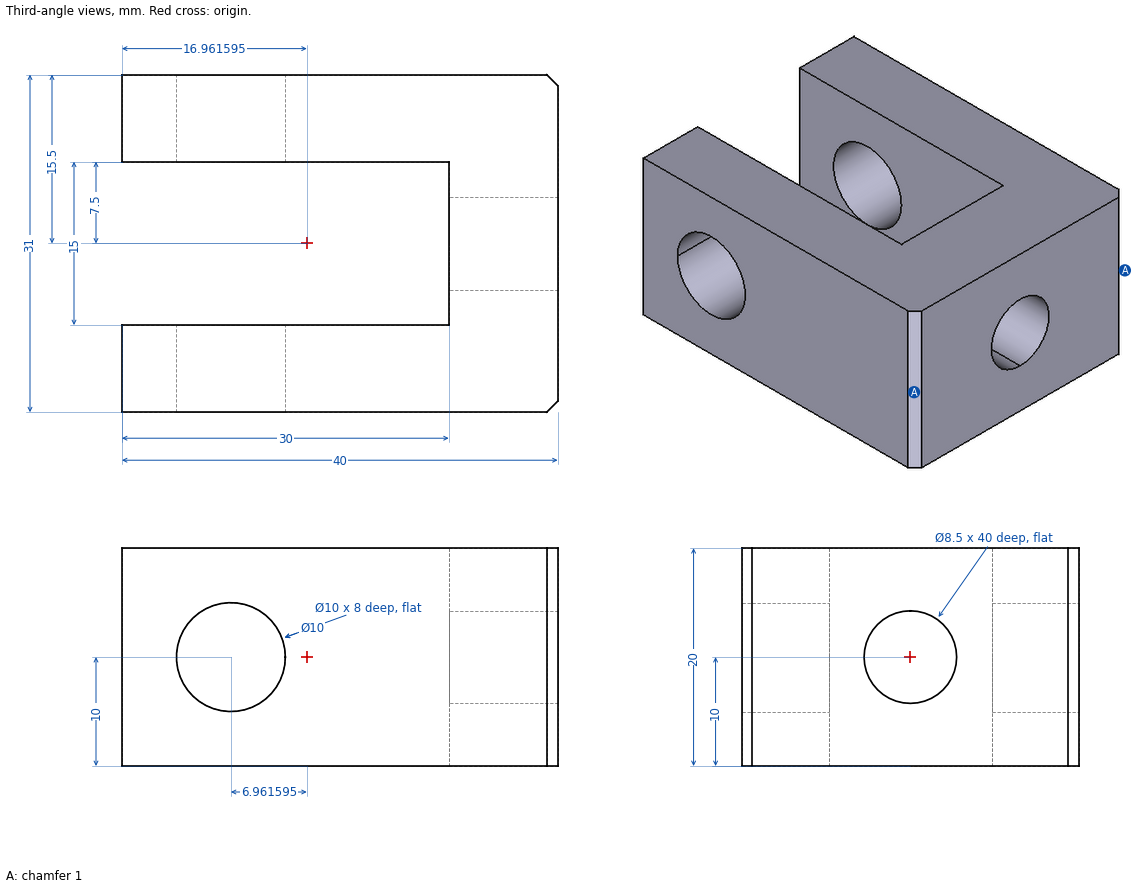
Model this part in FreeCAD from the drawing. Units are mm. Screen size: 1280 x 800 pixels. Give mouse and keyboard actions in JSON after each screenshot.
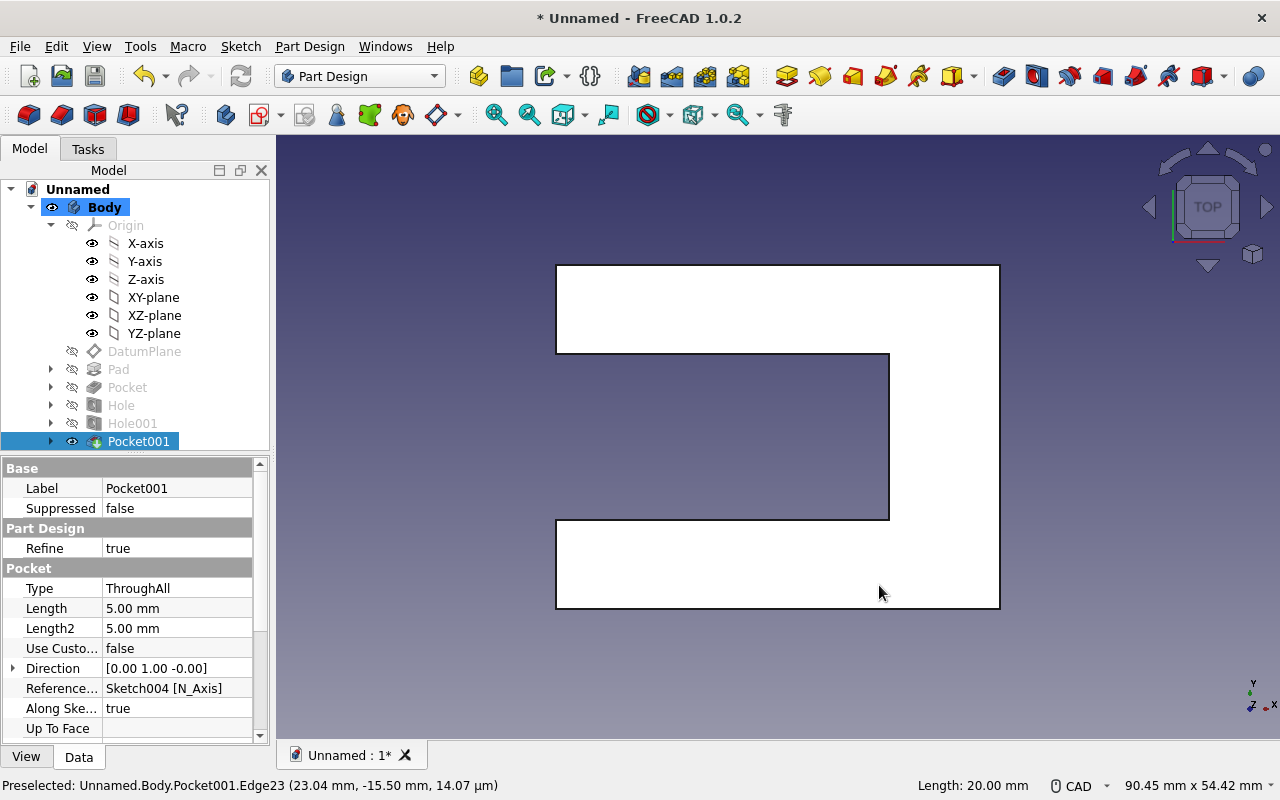
{"action": "key", "text": "1"}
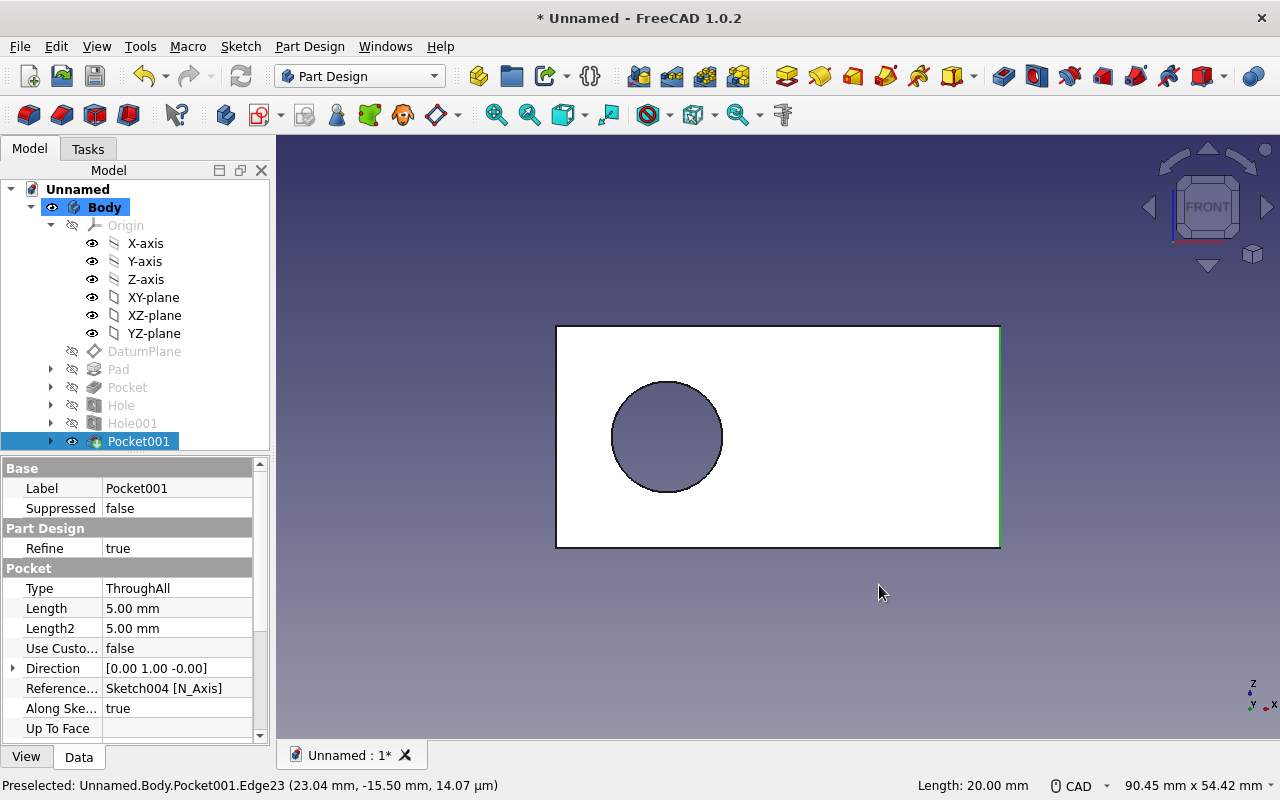
{"action": "left_click", "coordinate": [497, 116]}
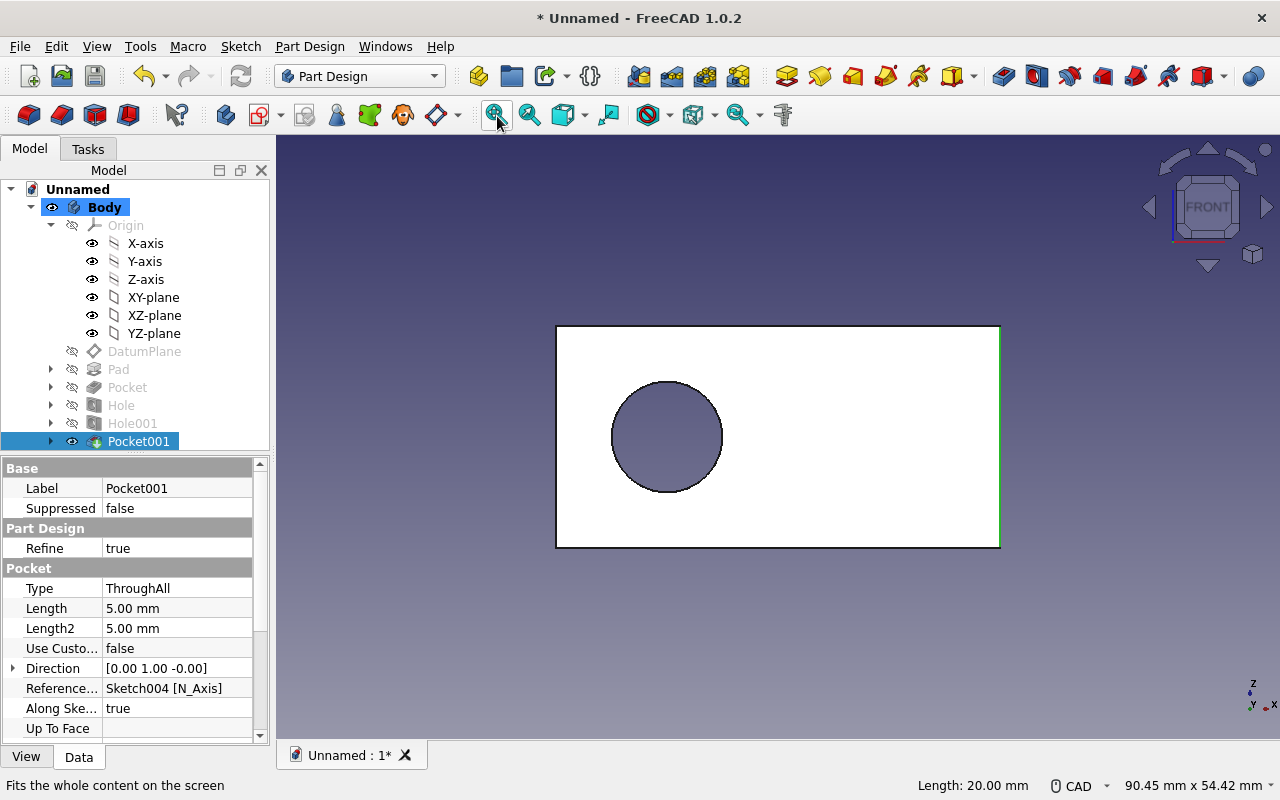
{"action": "key", "text": "3"}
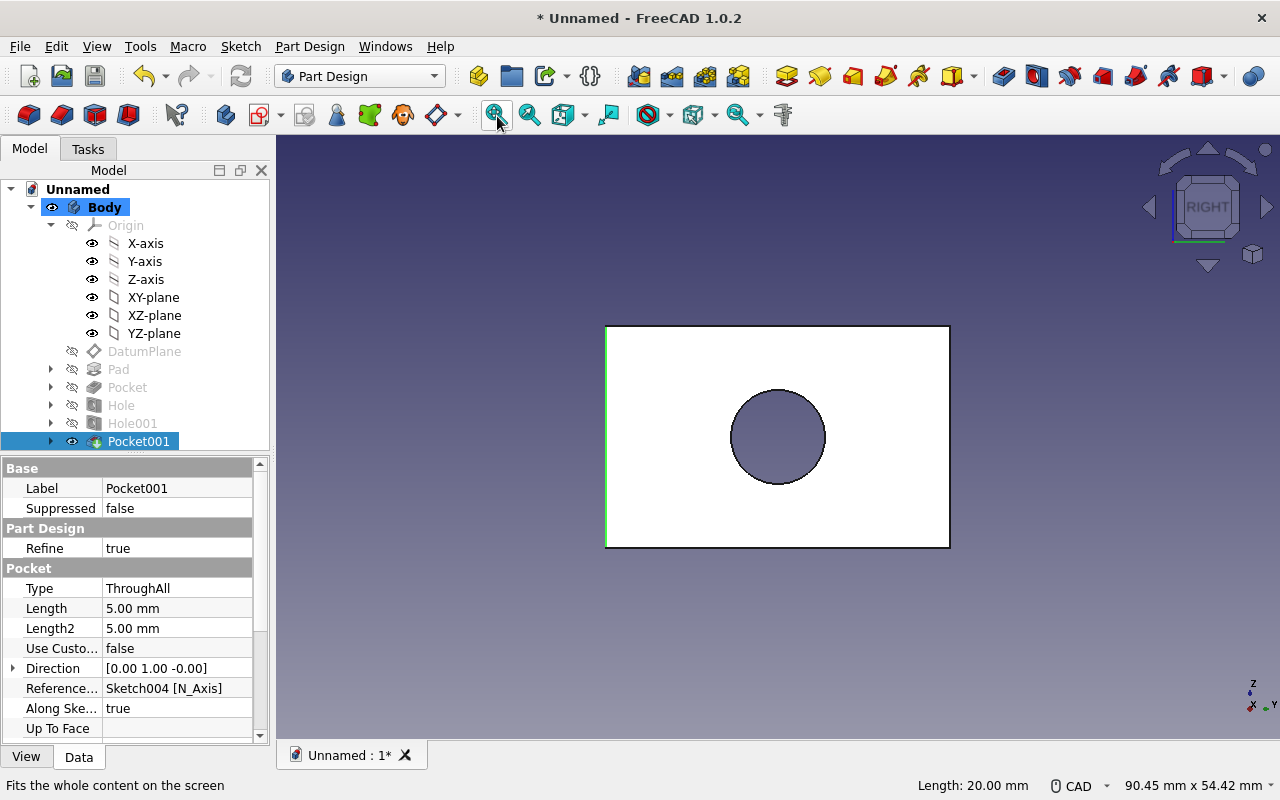
{"action": "key", "text": "v f"}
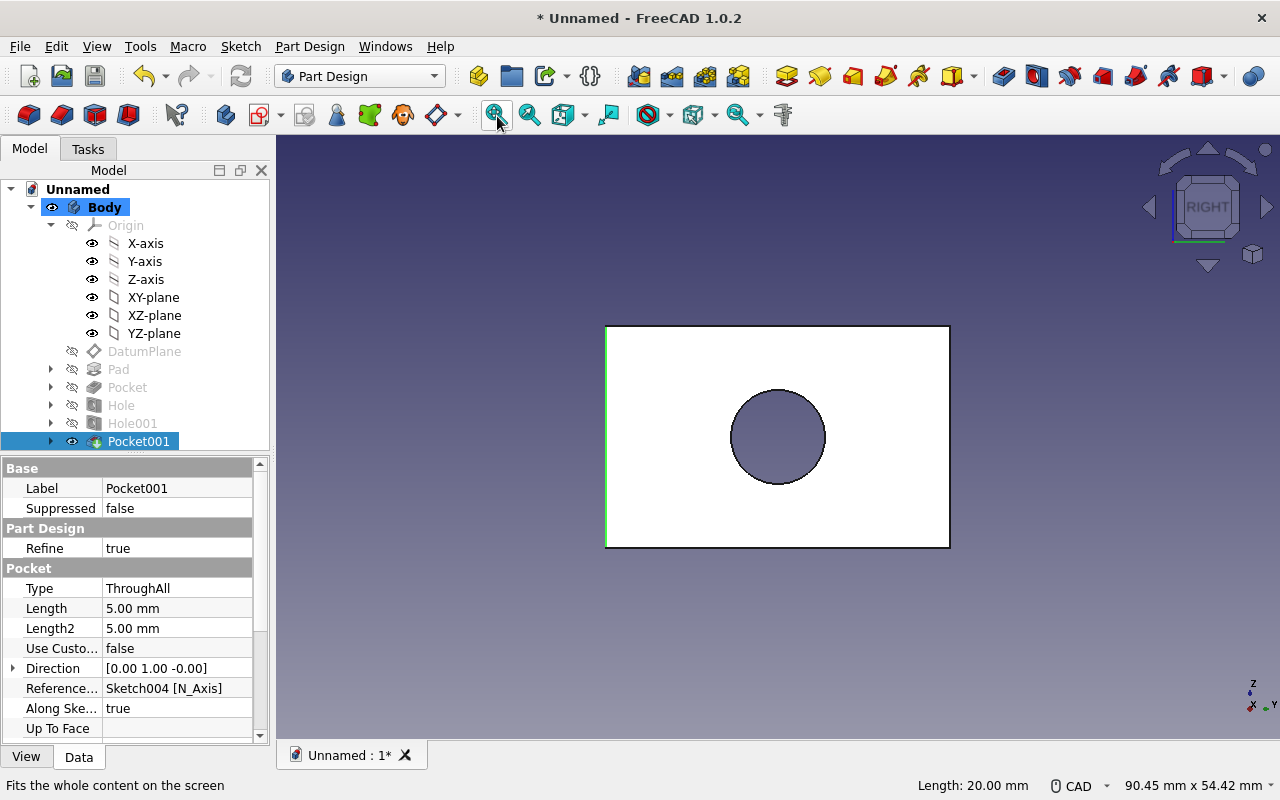
{"action": "left_click", "coordinate": [950, 436], "text": "ctrl"}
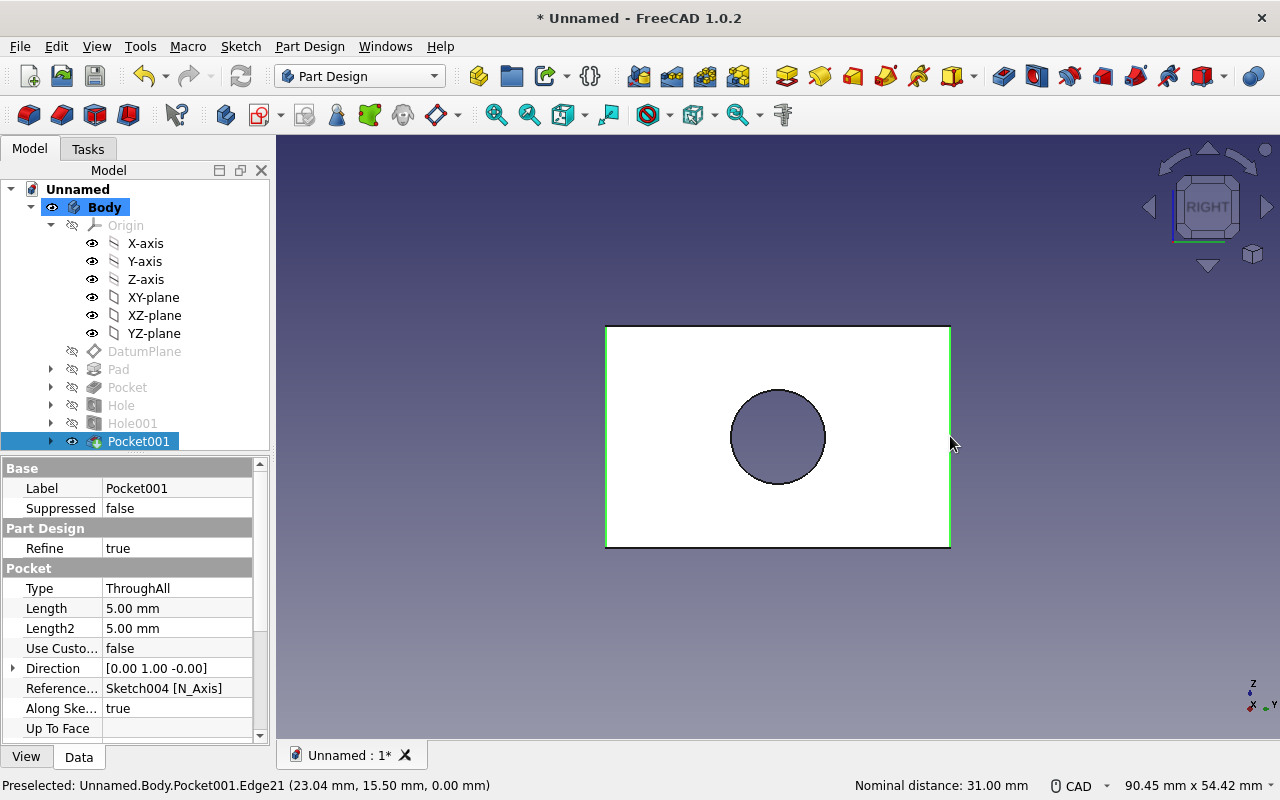
{"action": "left_click", "coordinate": [62, 116]}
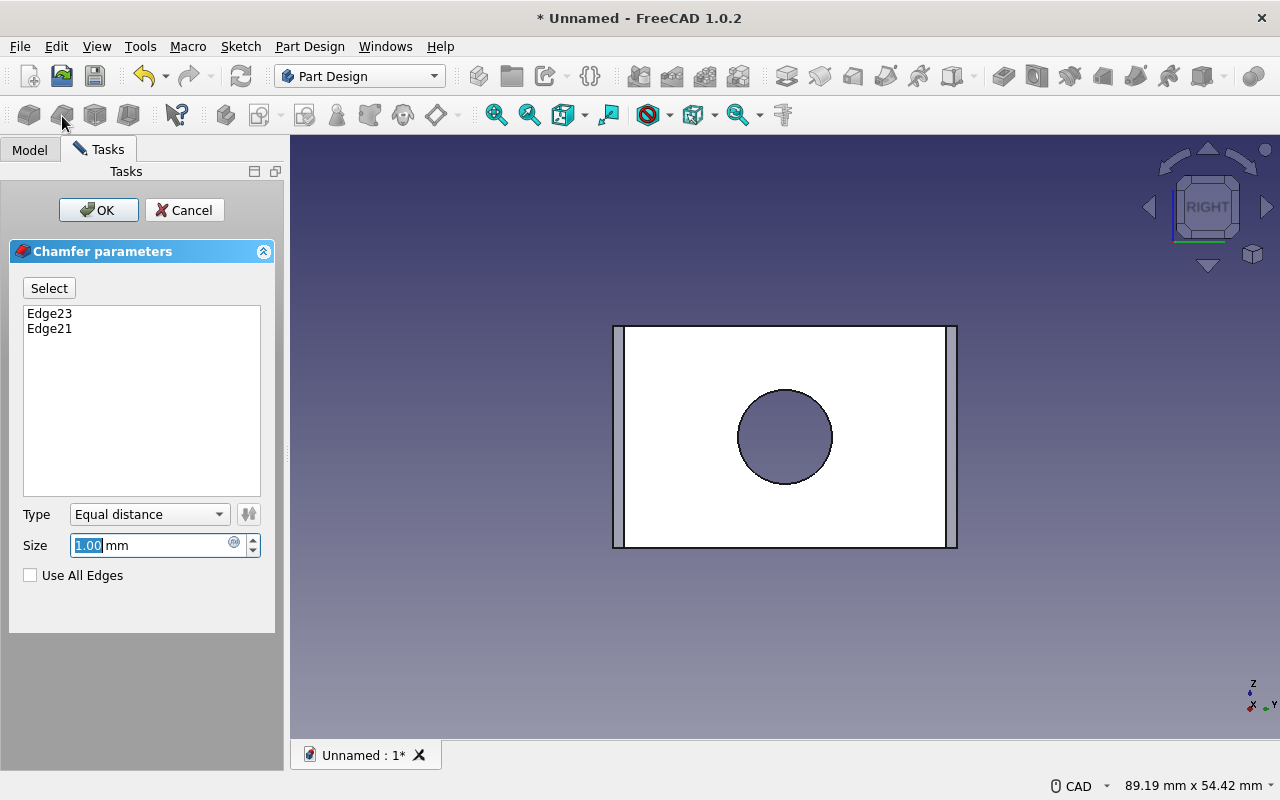
{"action": "type", "text": "1"}
{"action": "key", "text": "Tab"}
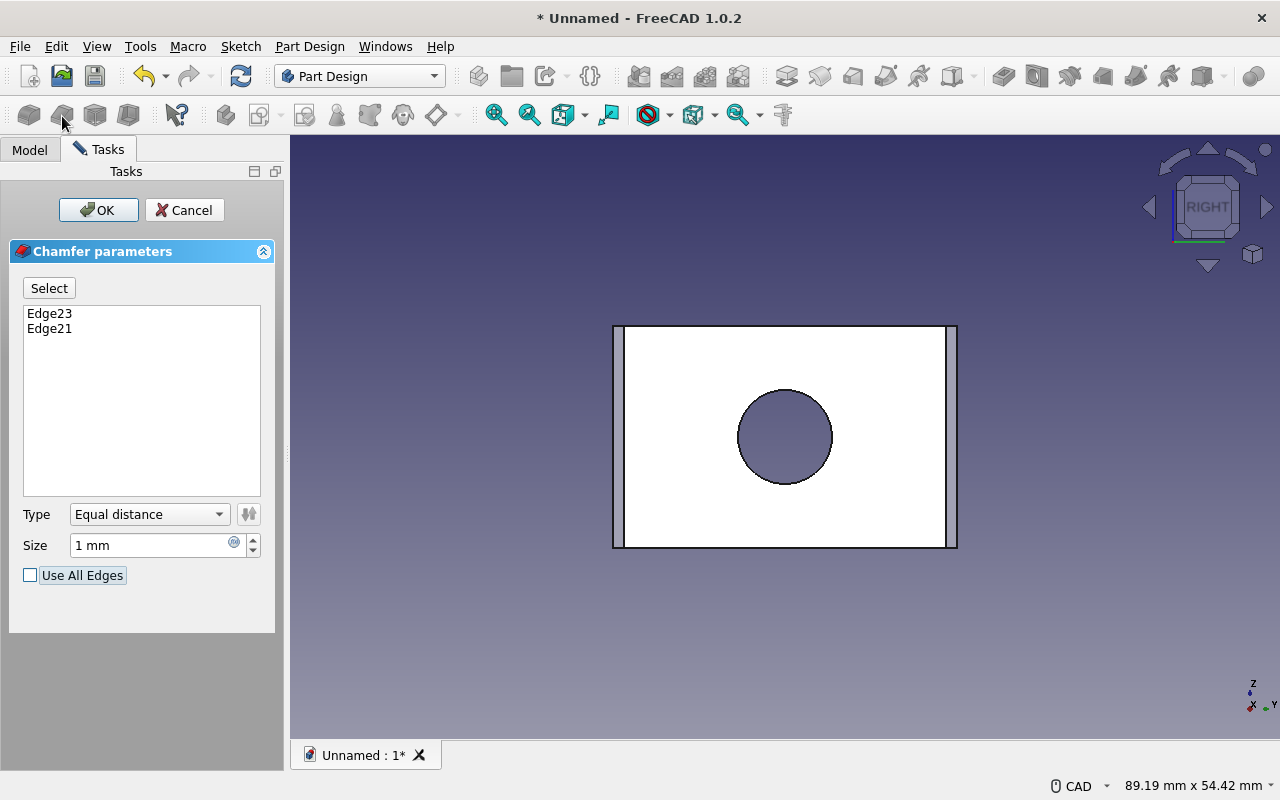
{"action": "left_click", "coordinate": [99, 210]}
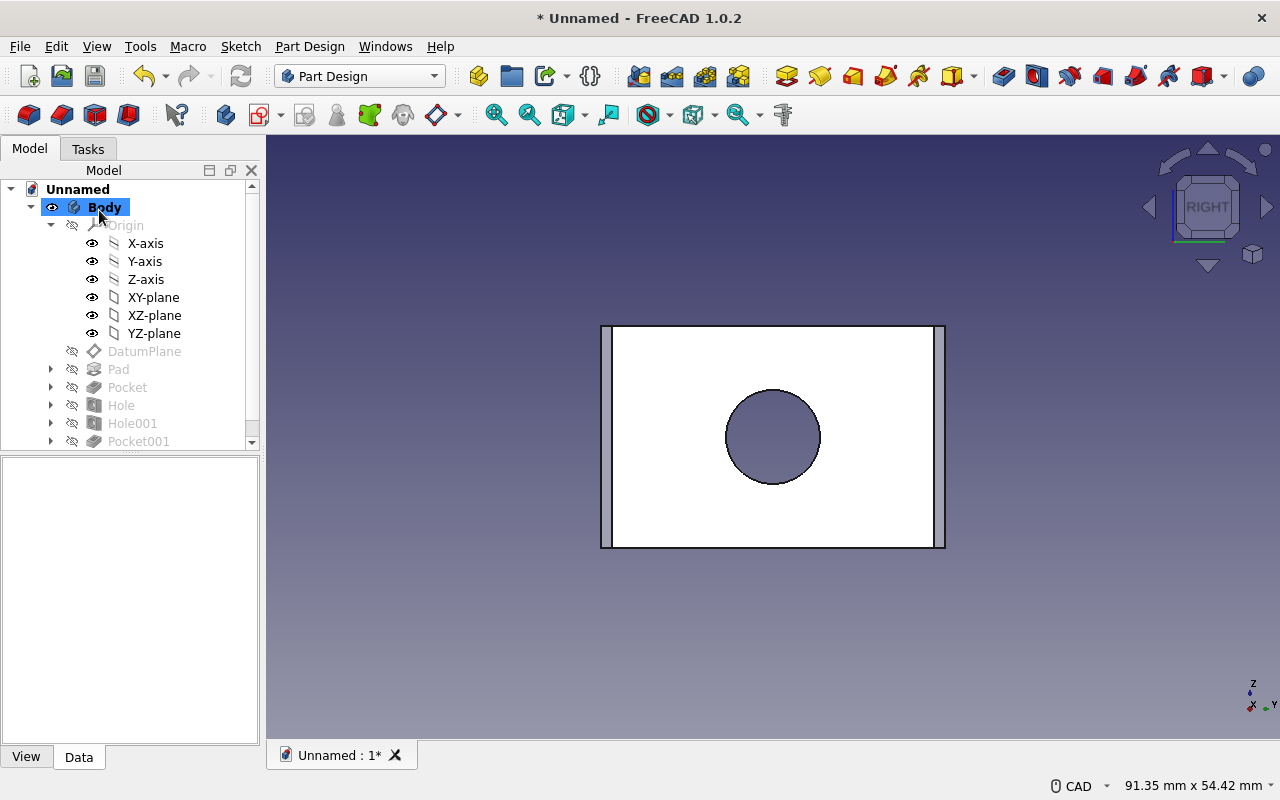
{"action": "key", "text": "0"}